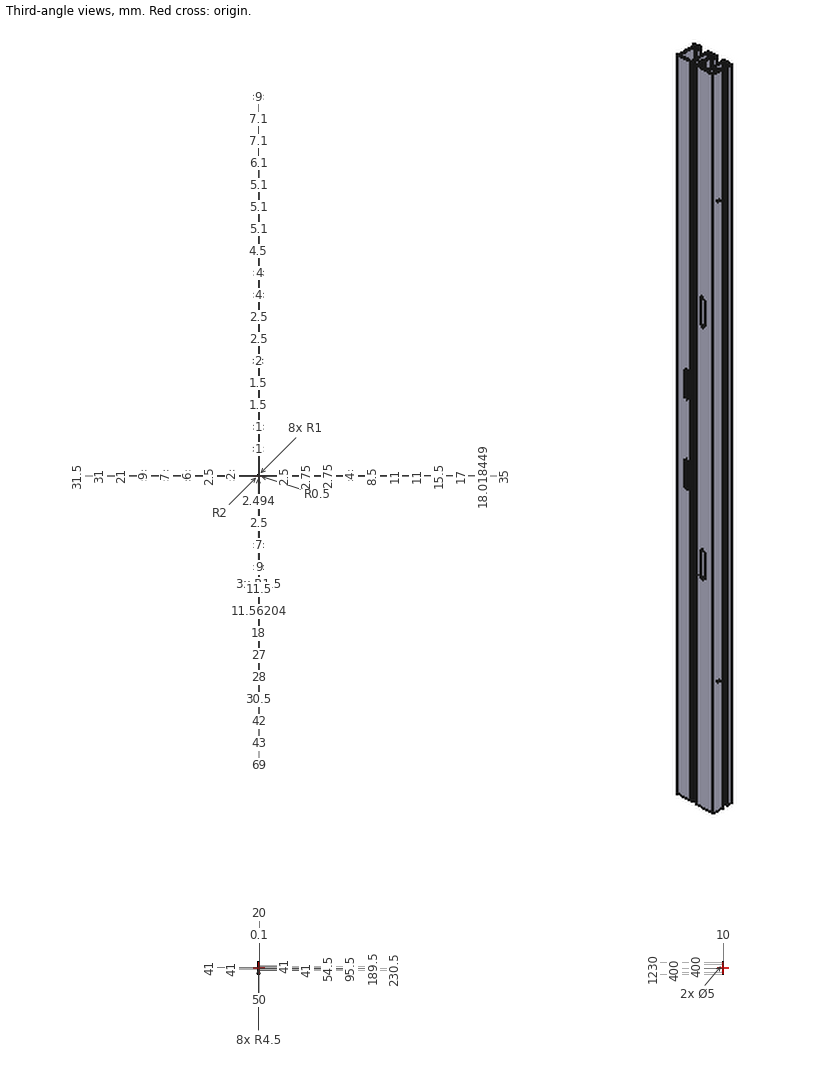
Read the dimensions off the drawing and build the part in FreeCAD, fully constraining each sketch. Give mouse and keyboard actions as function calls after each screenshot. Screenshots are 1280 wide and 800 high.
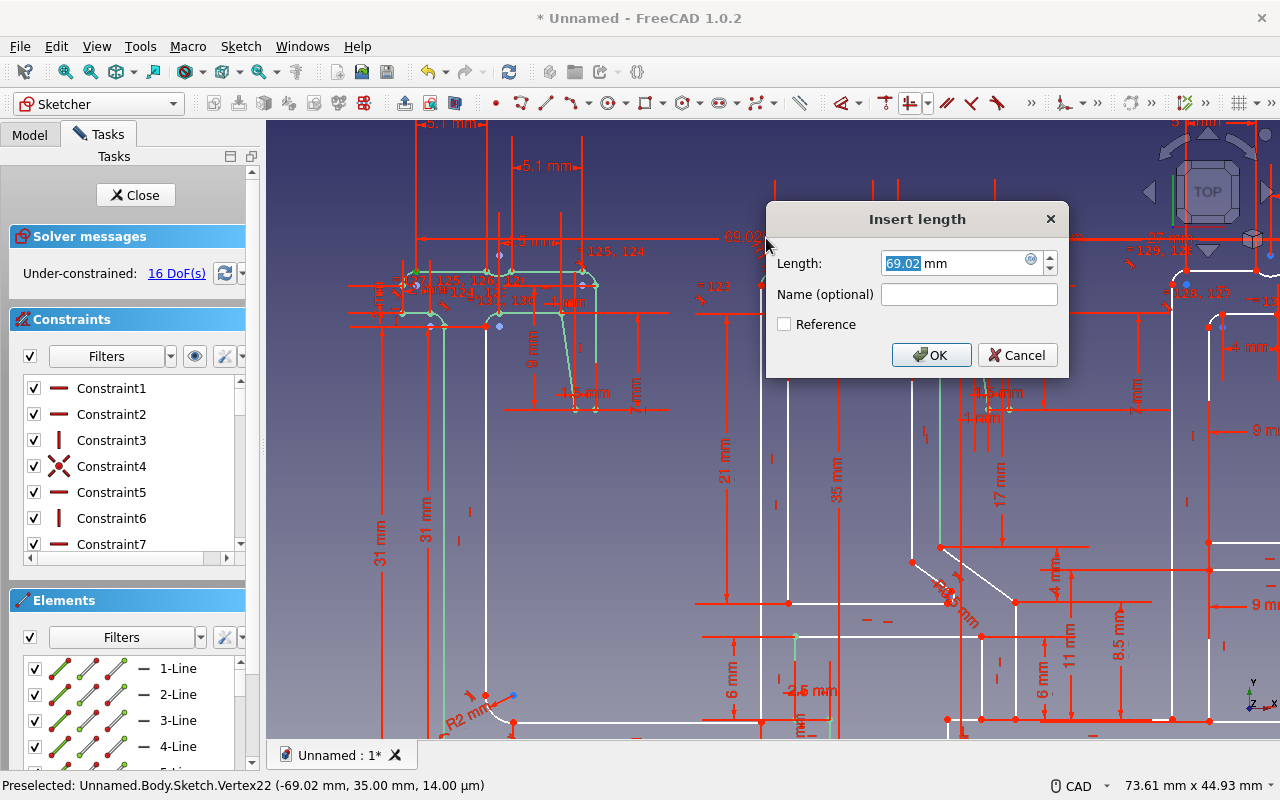
text(69)
key(Return)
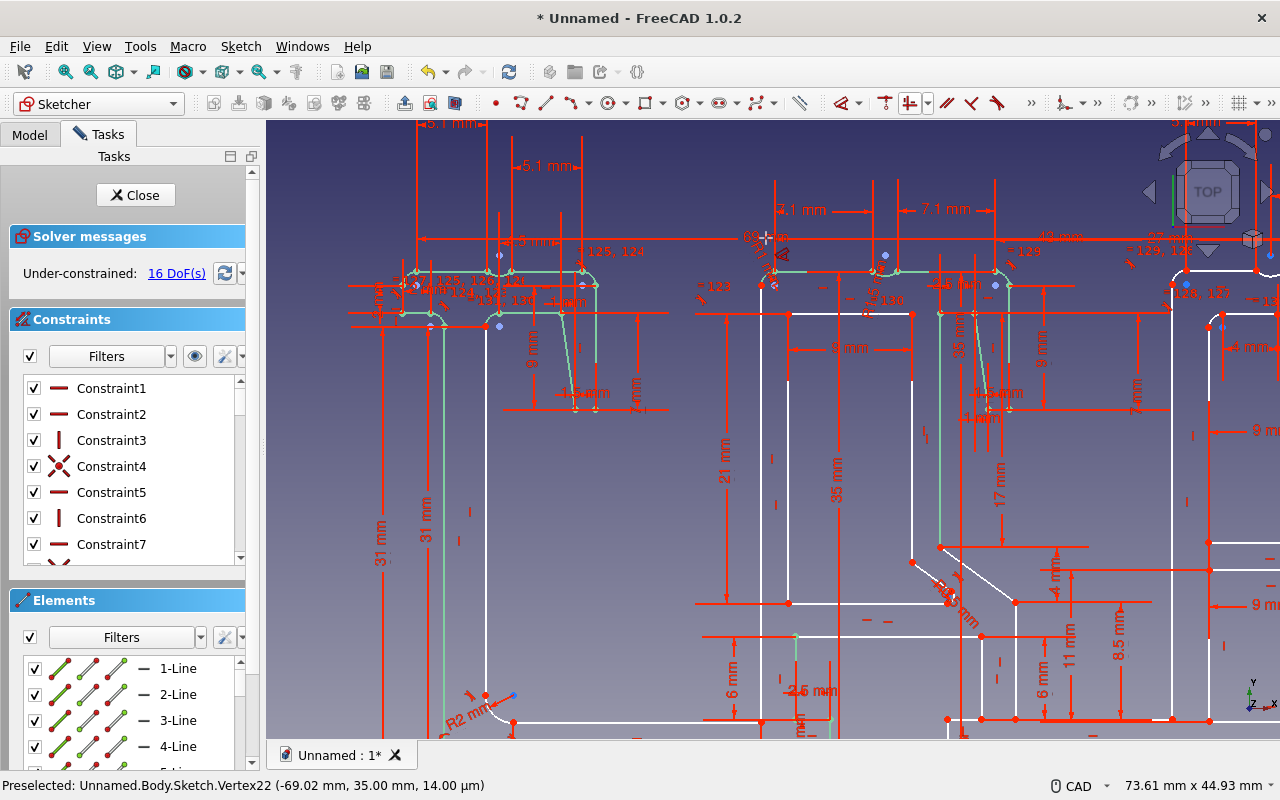
scroll(485, 328, down, 3)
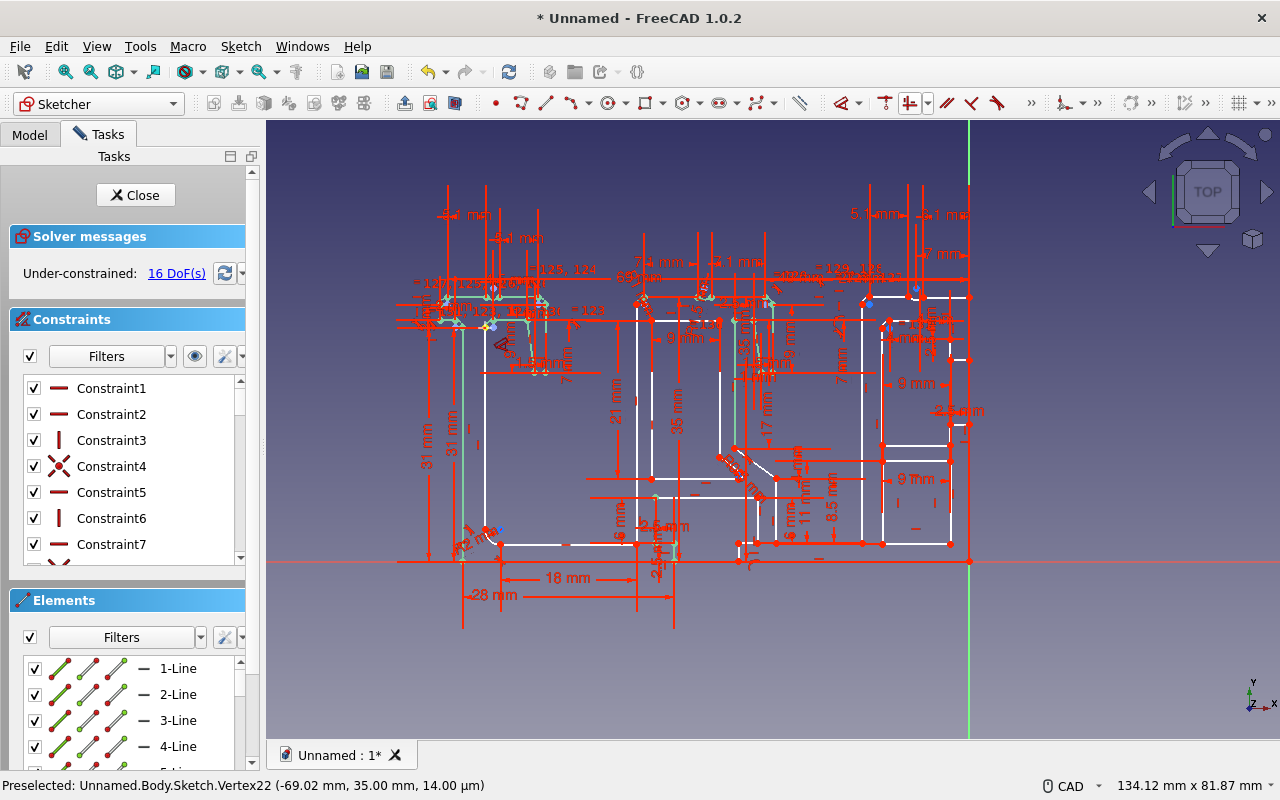
scroll(882, 328, up, 3)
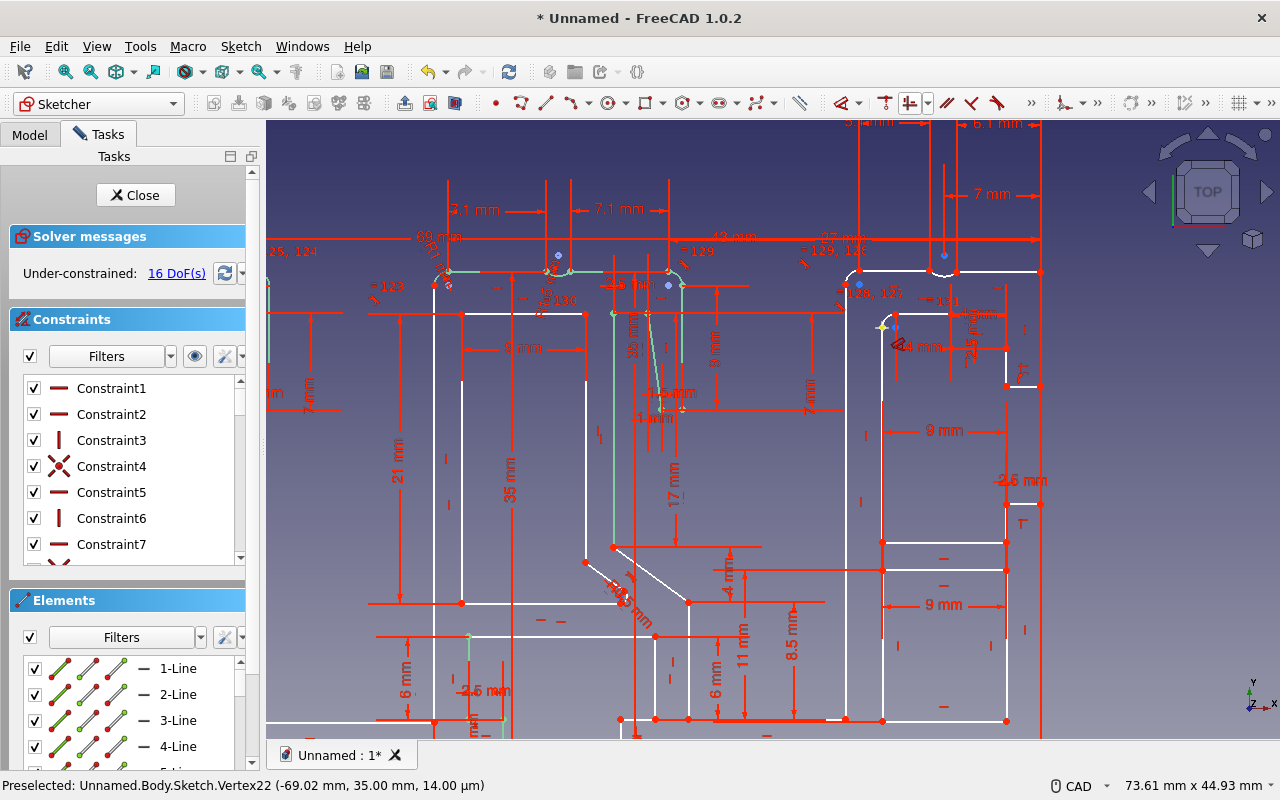
click(882, 328)
click(1075, 519)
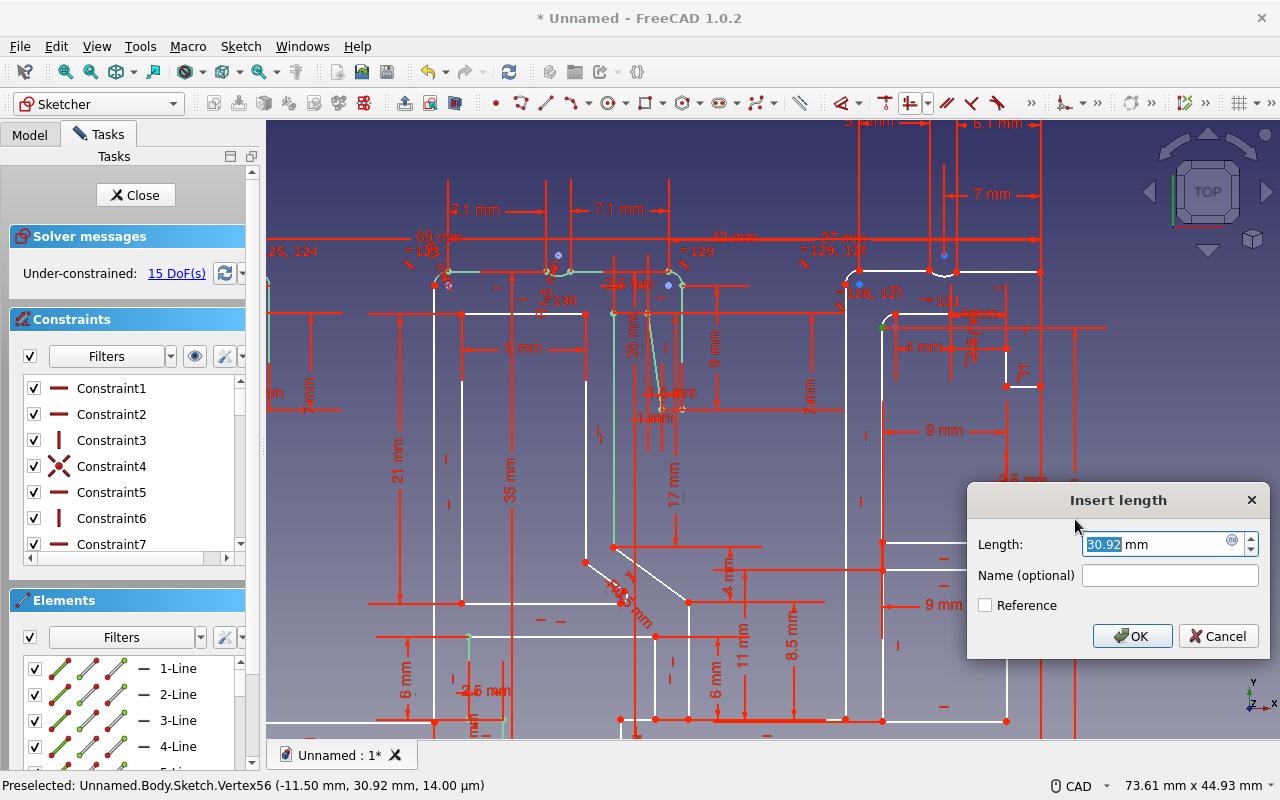
text(31)
key(Return)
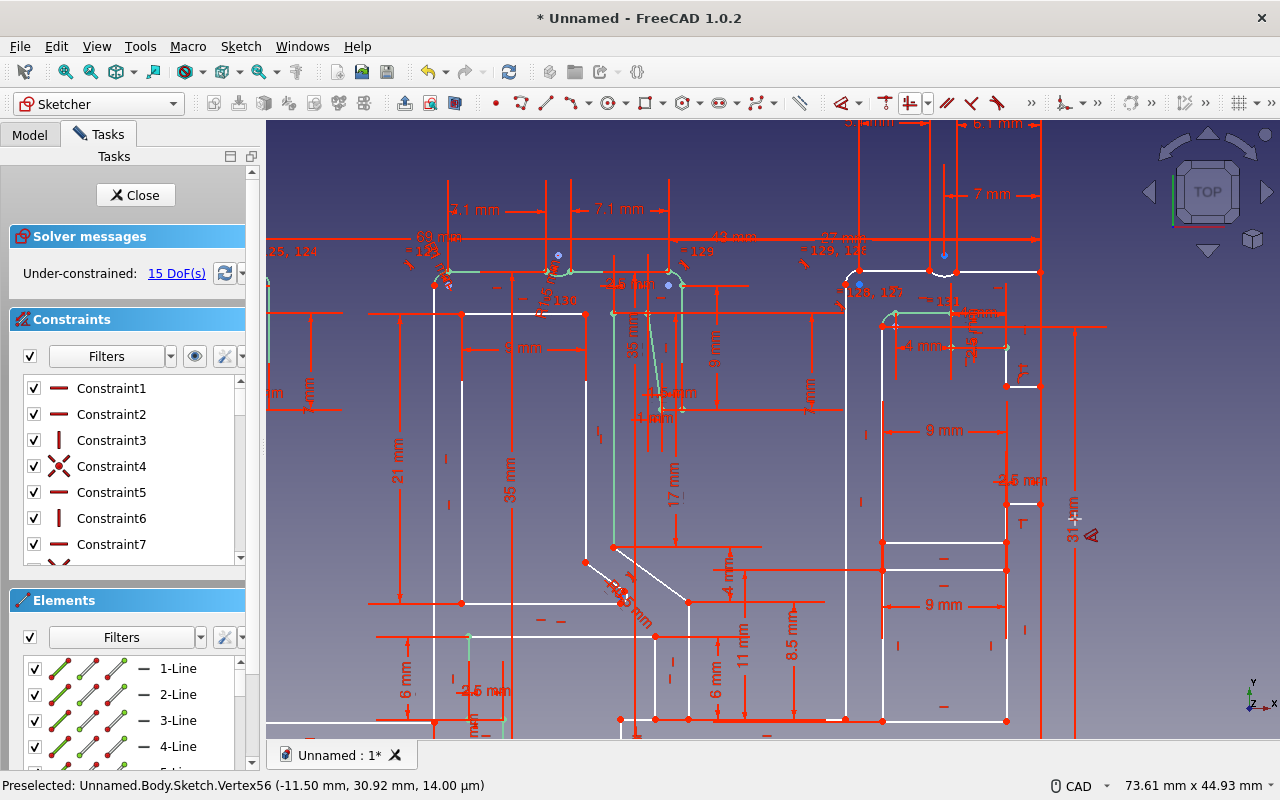
click(1041, 272)
click(1075, 391)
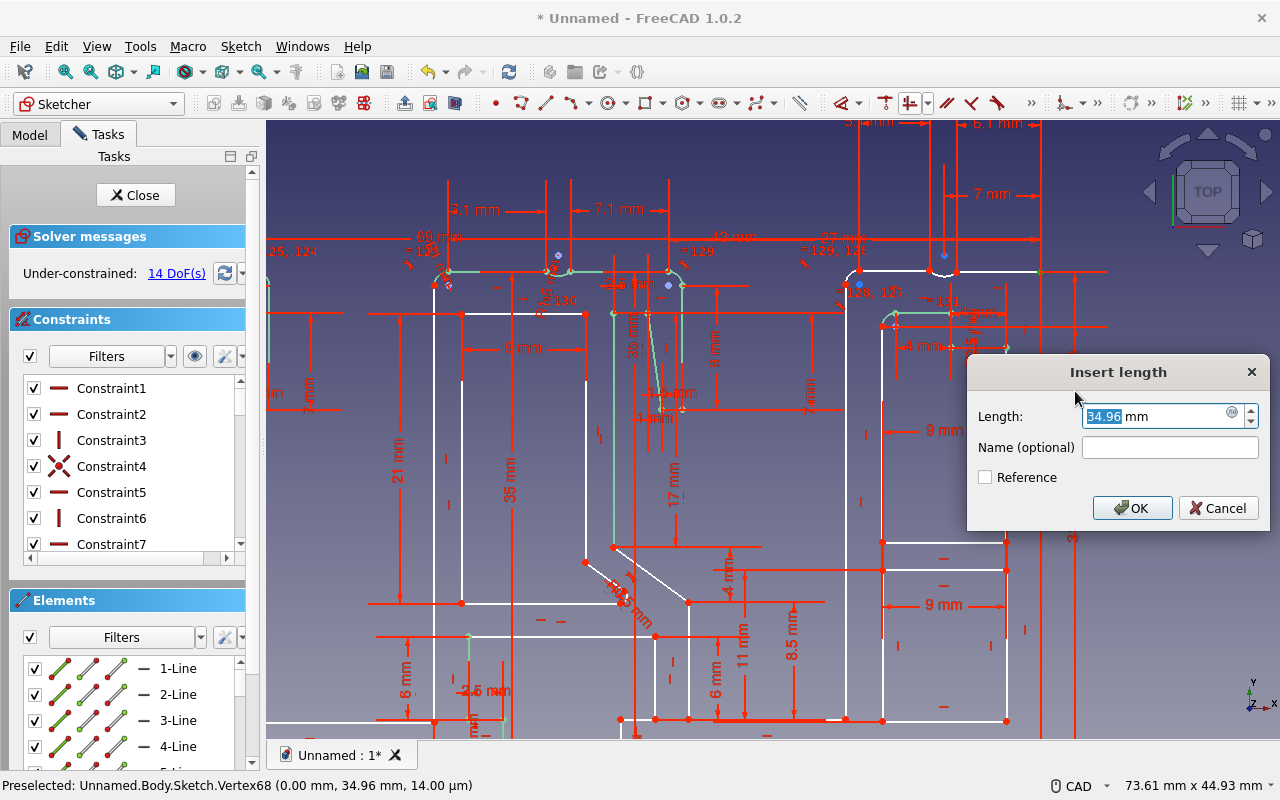
text(35)
key(Return)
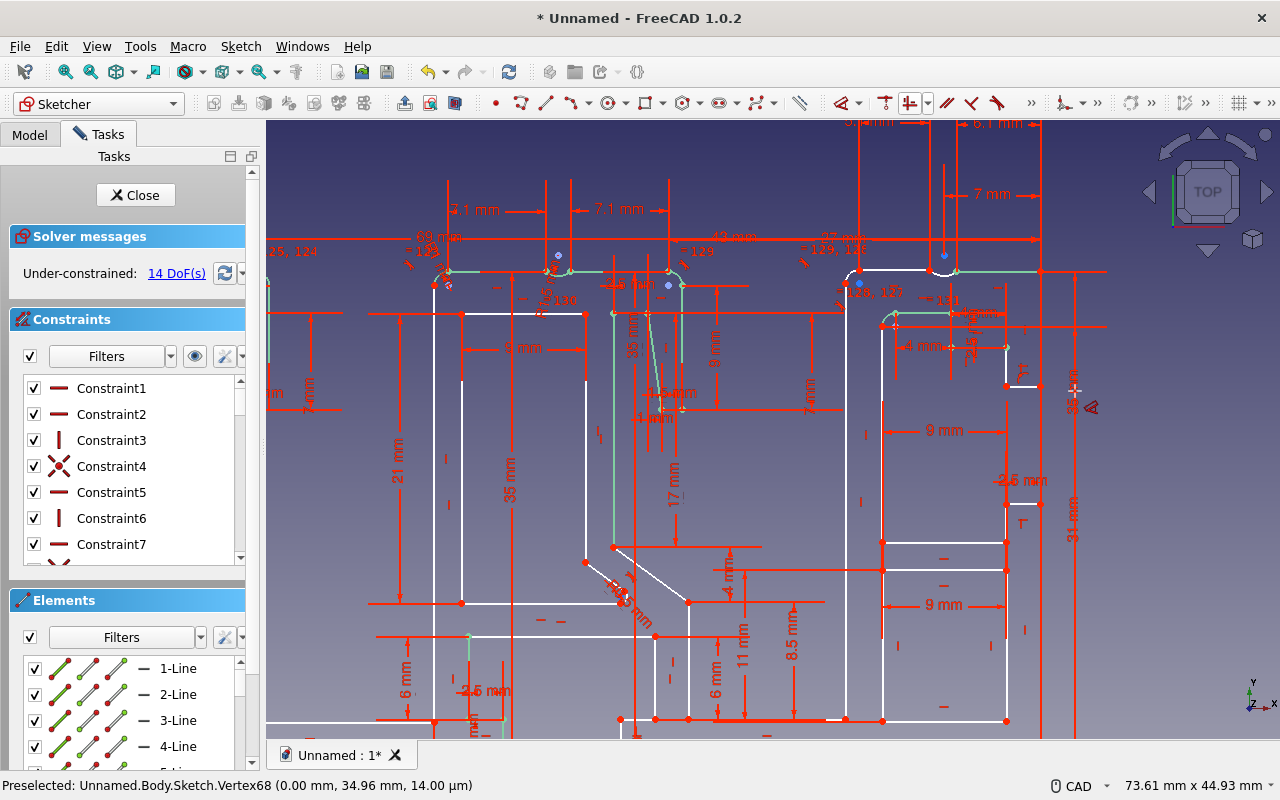
click(930, 270)
click(1075, 592)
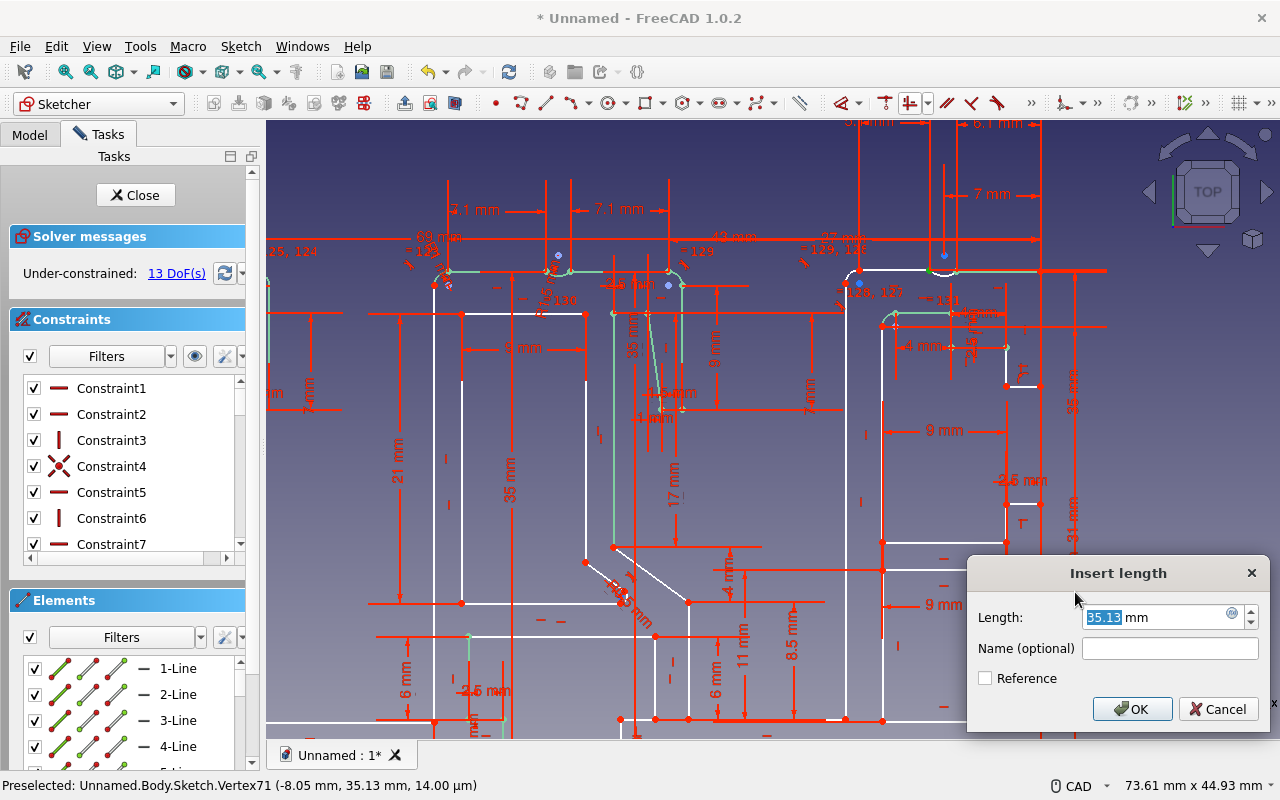
text(35)
key(Return)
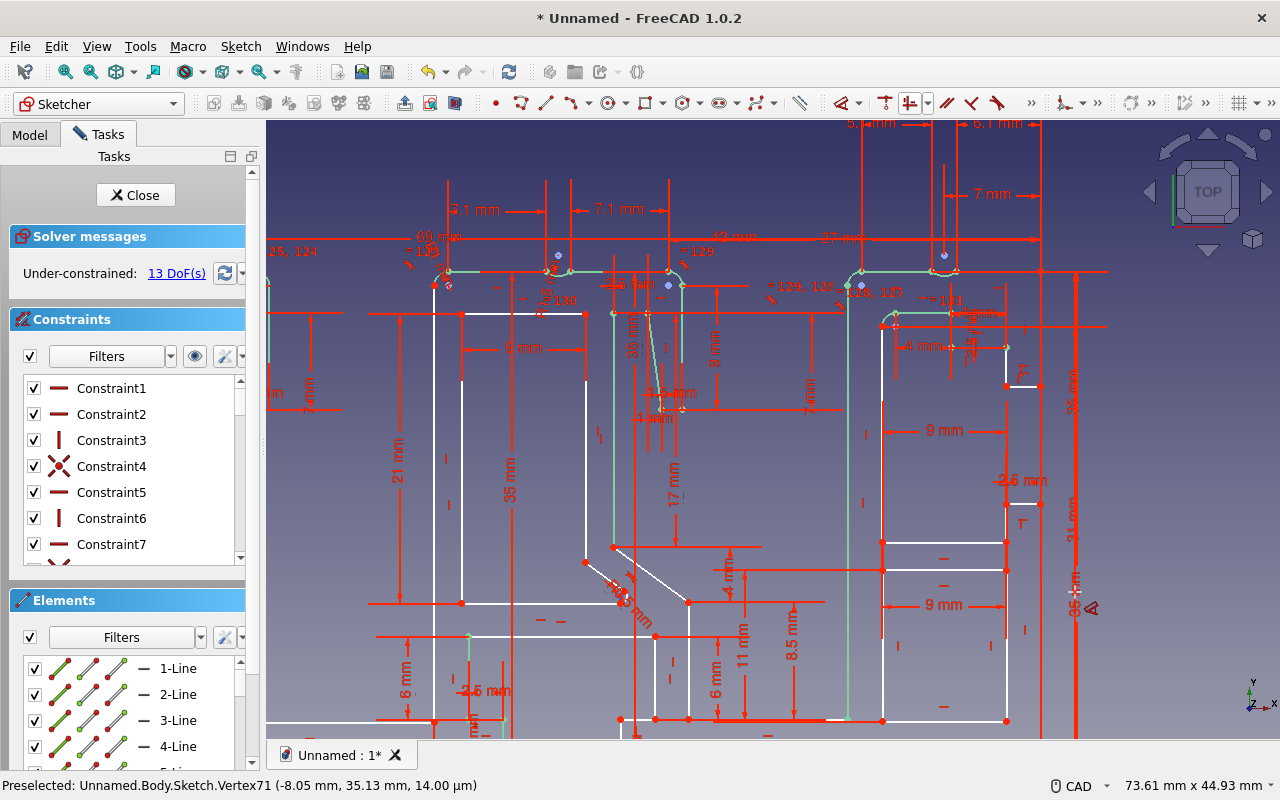
scroll(620, 604, up, 3)